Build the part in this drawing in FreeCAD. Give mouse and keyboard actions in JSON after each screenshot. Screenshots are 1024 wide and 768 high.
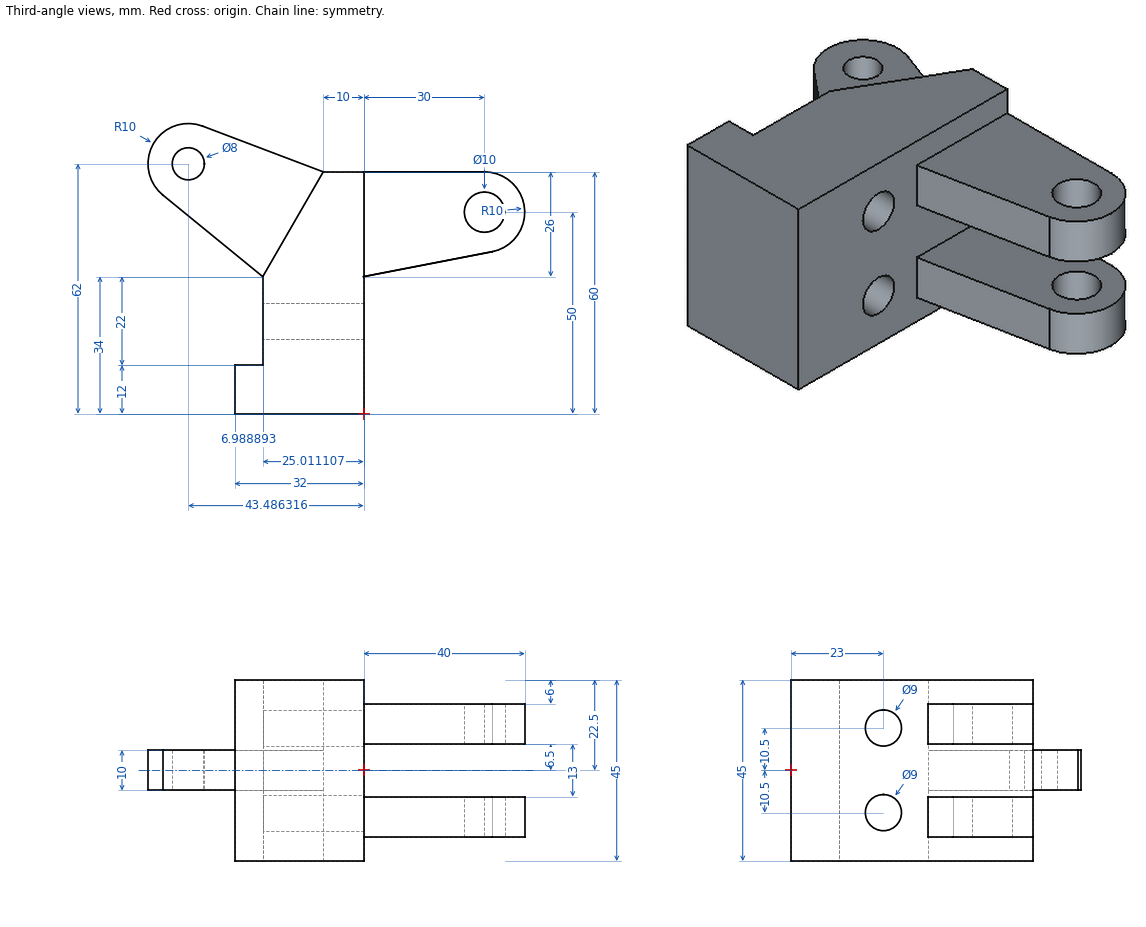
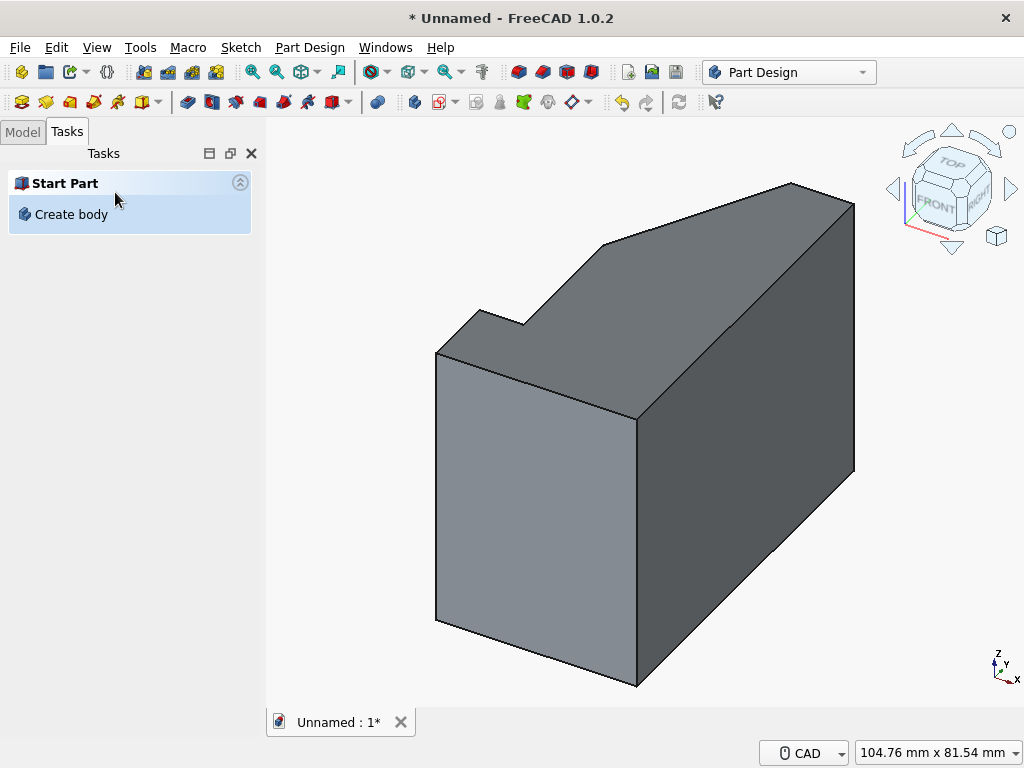
{"action": "left_click", "coordinate": [440, 102]}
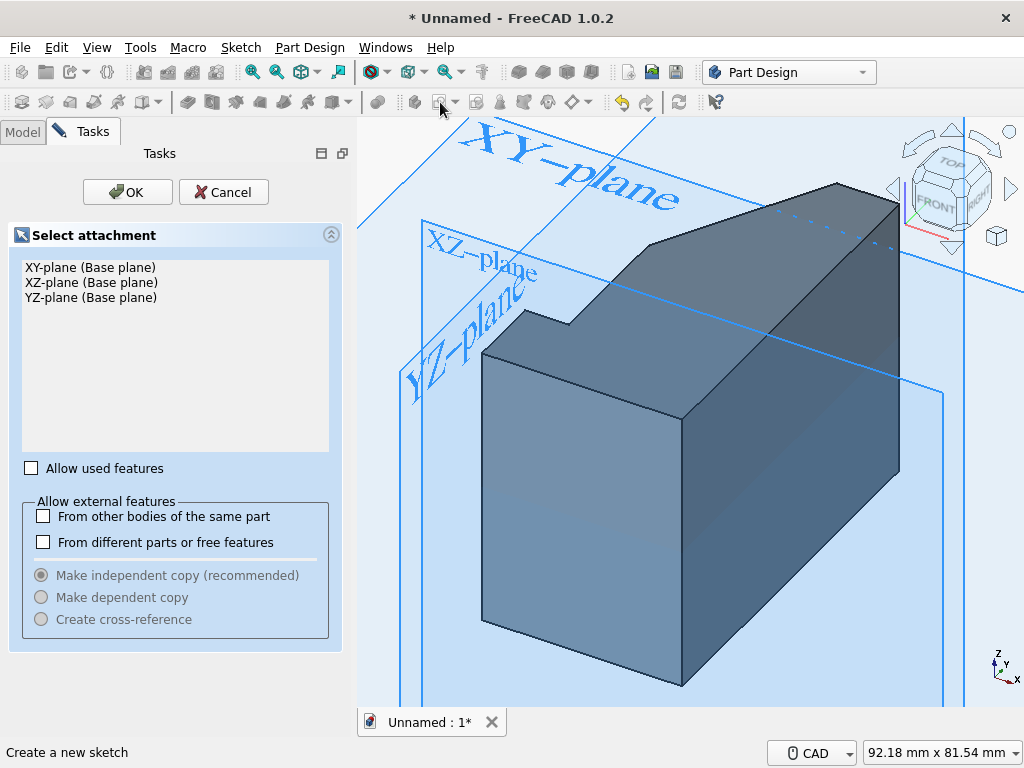
{"action": "left_click", "coordinate": [82, 268]}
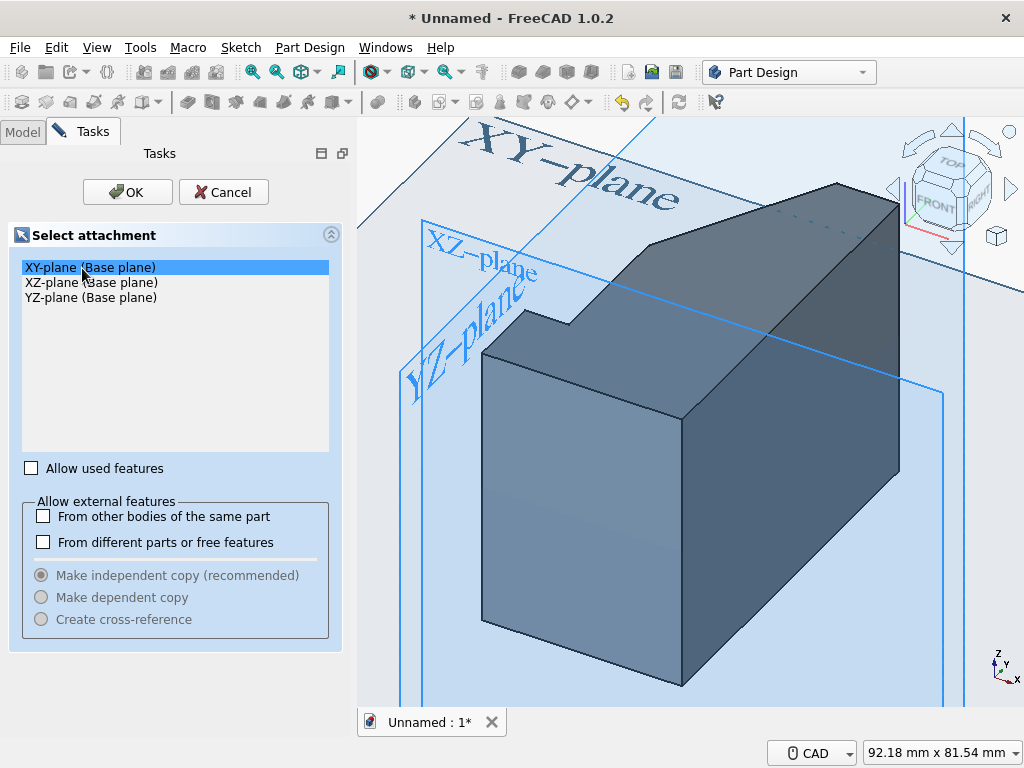
{"action": "left_click", "coordinate": [128, 192]}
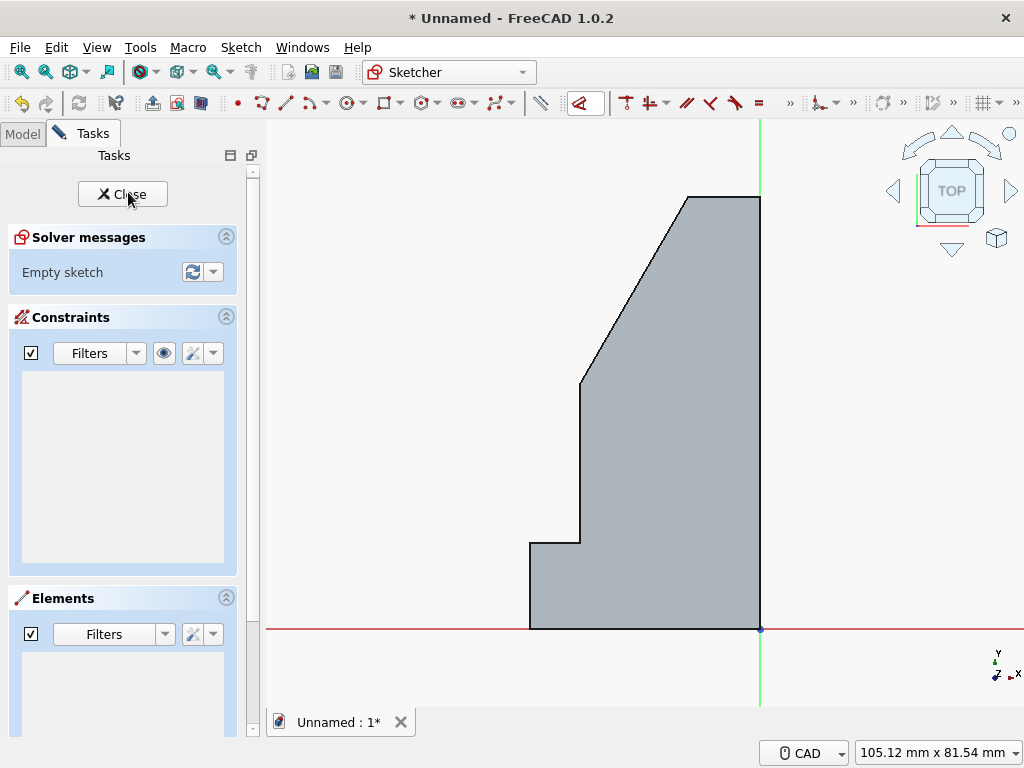
{"action": "left_click", "coordinate": [202, 104]}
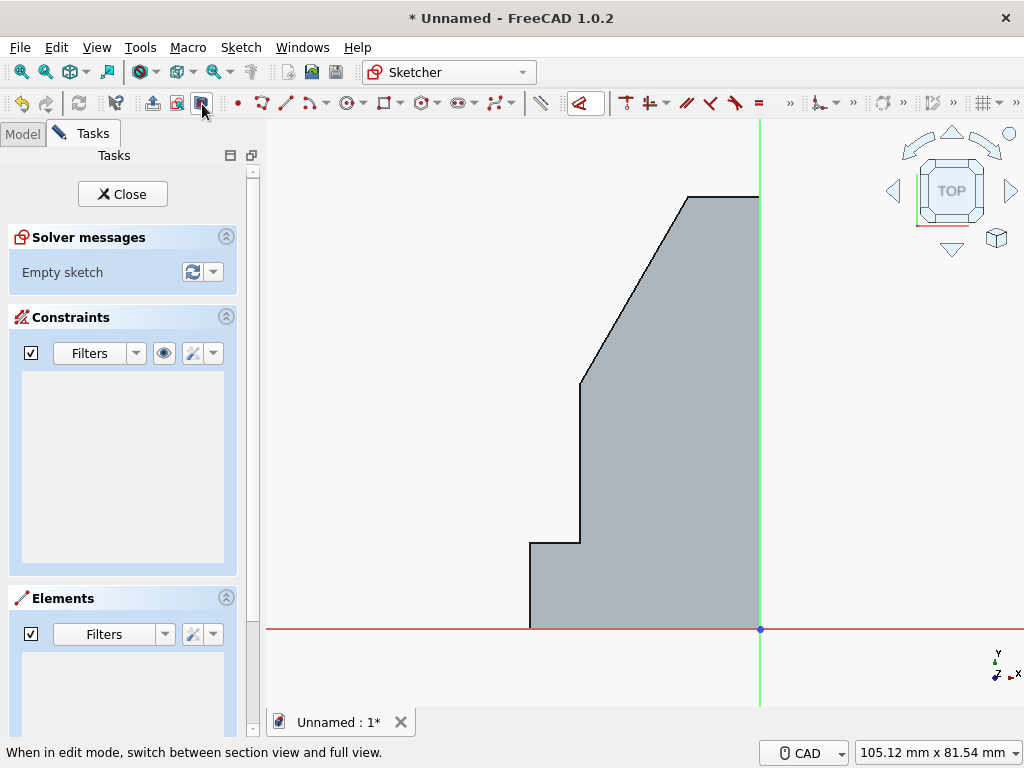
{"action": "scroll", "coordinate": [585, 496], "scroll_direction": "down", "scroll_amount": 2}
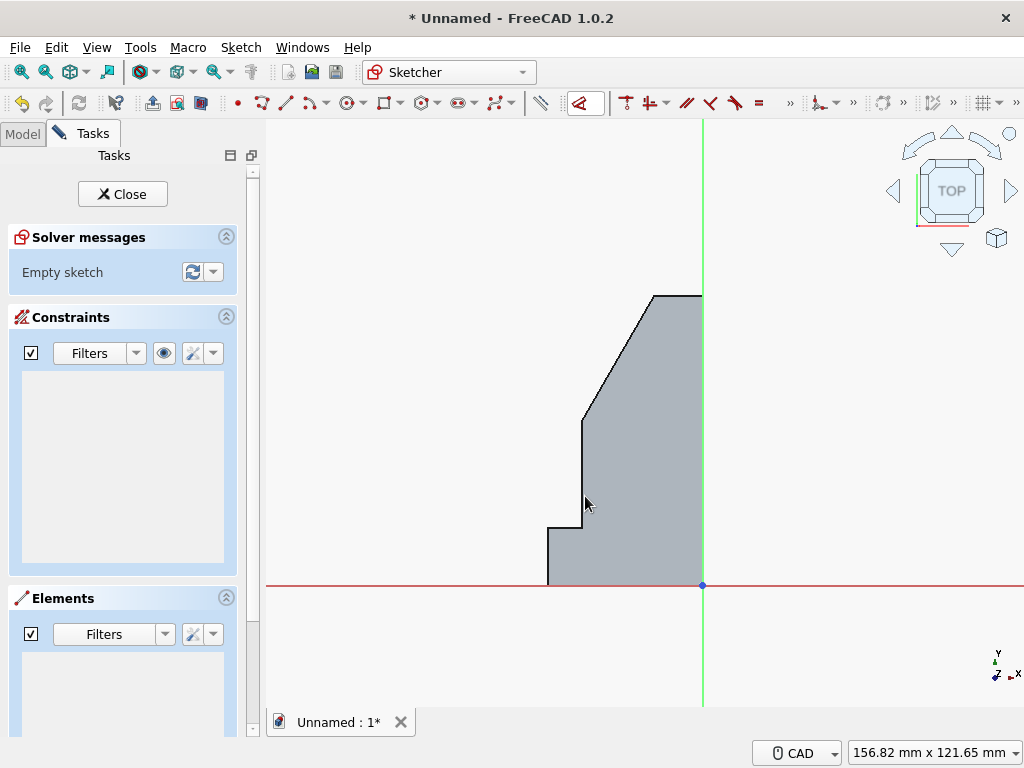
{"action": "key", "text": "g m"}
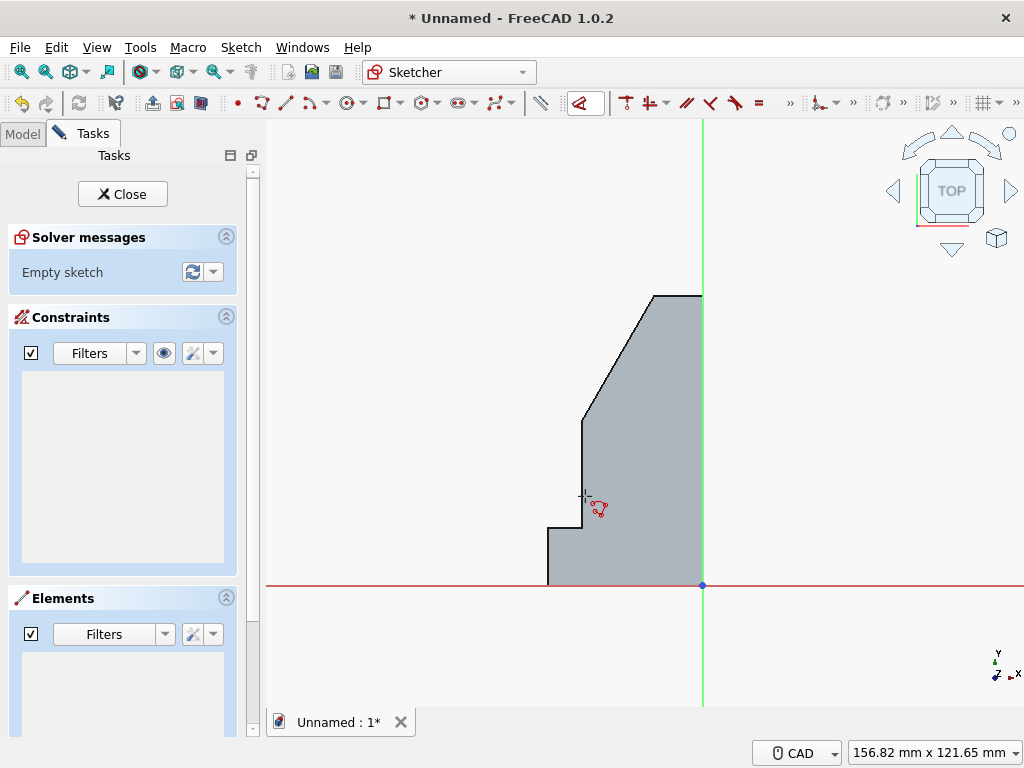
{"action": "left_click", "coordinate": [462, 323]}
{"action": "left_click", "coordinate": [582, 421]}
{"action": "left_click", "coordinate": [654, 296]}
{"action": "left_click", "coordinate": [510, 241]}
{"action": "right_click", "coordinate": [510, 241]}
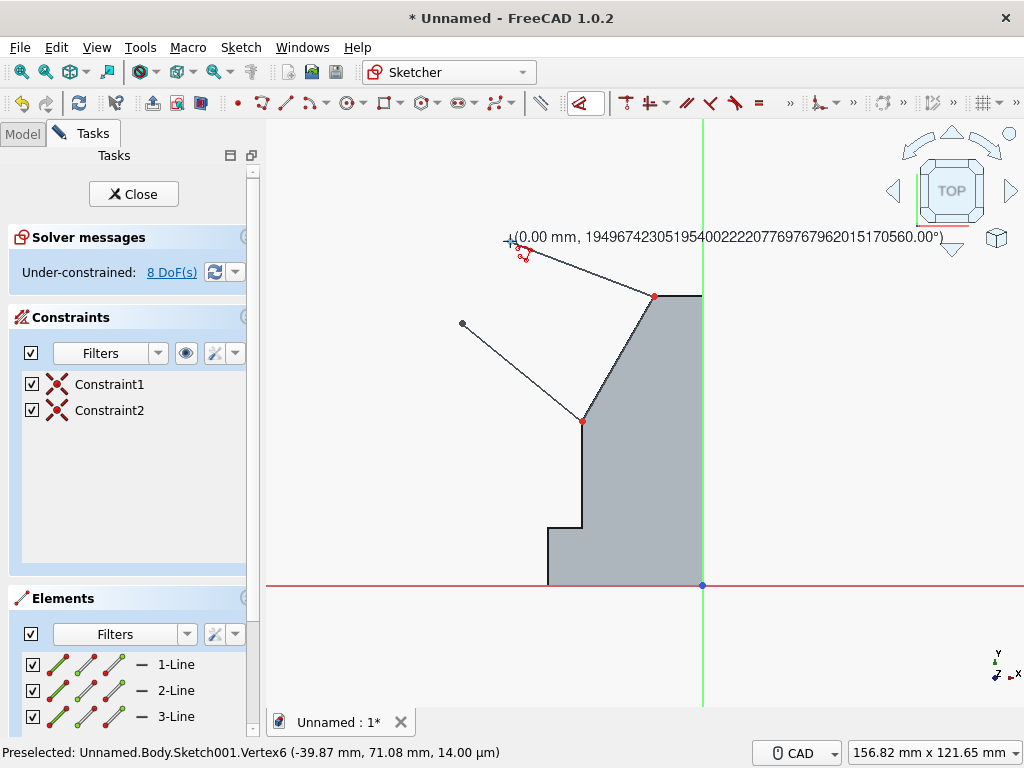
{"action": "key", "text": "g 3 a"}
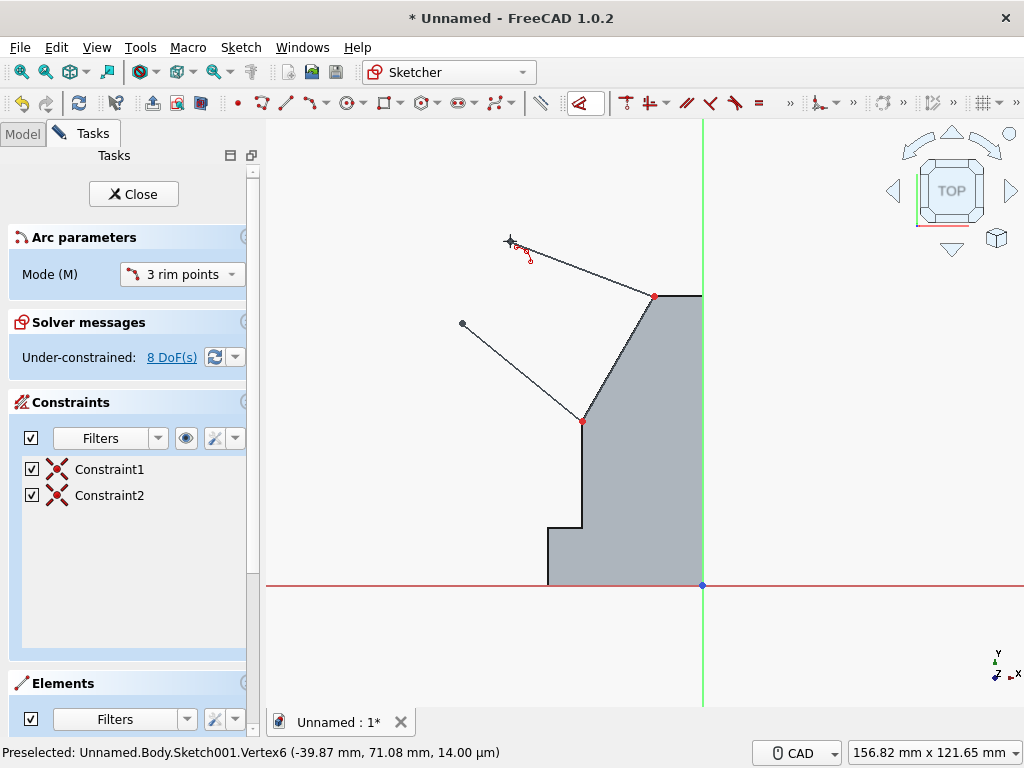
{"action": "left_click", "coordinate": [510, 242]}
{"action": "left_click", "coordinate": [462, 324]}
{"action": "left_click", "coordinate": [451, 262]}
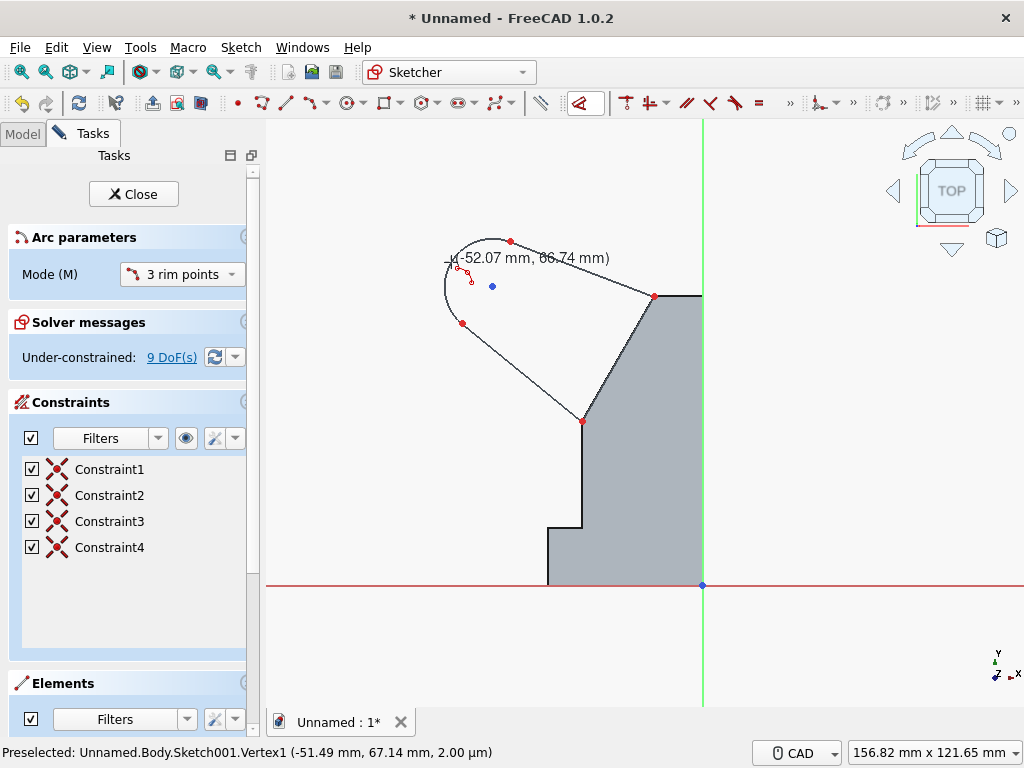
{"action": "key", "text": "g c"}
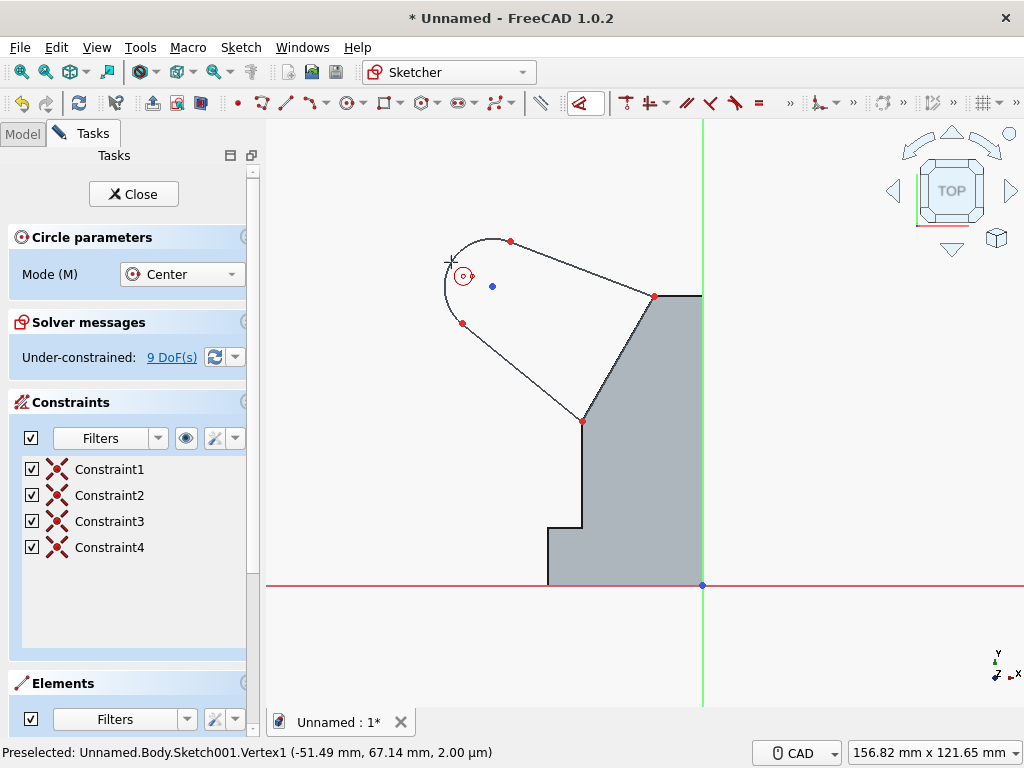
{"action": "left_click", "coordinate": [492, 286]}
{"action": "mouse_move", "coordinate": [506, 272]}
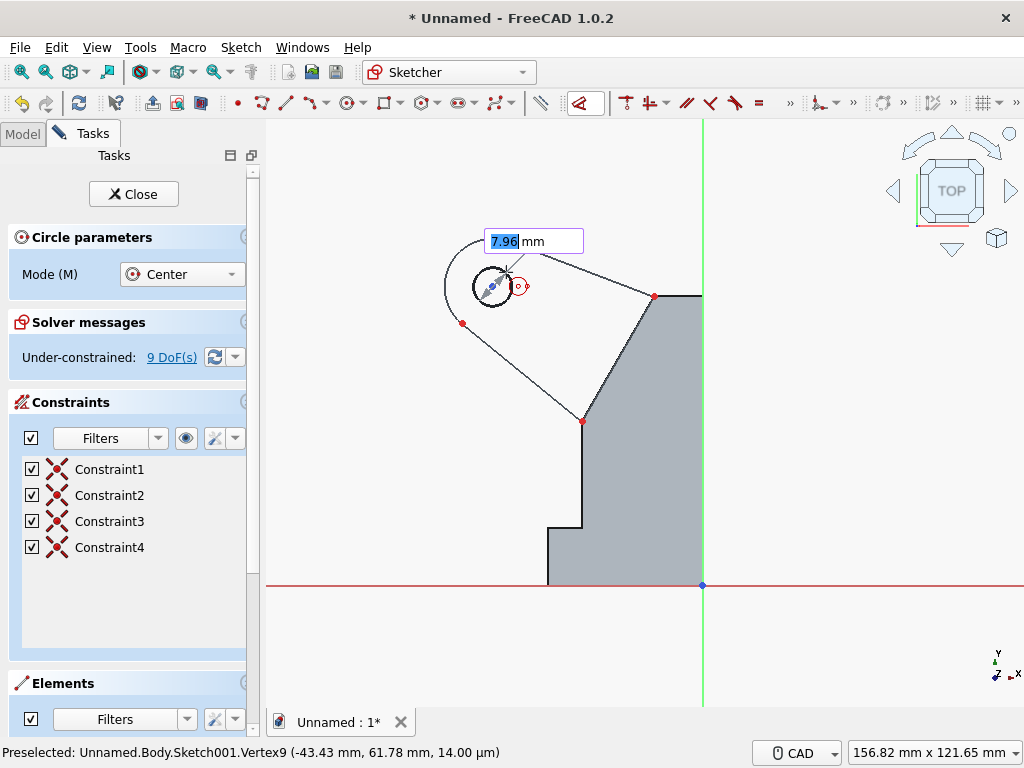
{"action": "type", "text": "8"}
{"action": "key", "text": "Return"}
{"action": "key", "text": "Escape"}